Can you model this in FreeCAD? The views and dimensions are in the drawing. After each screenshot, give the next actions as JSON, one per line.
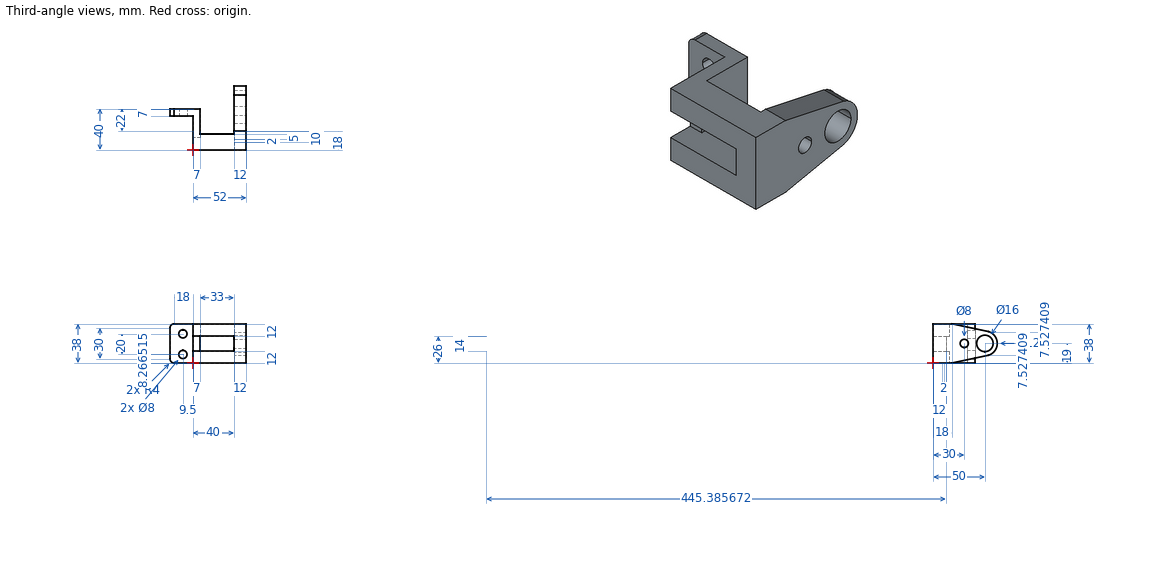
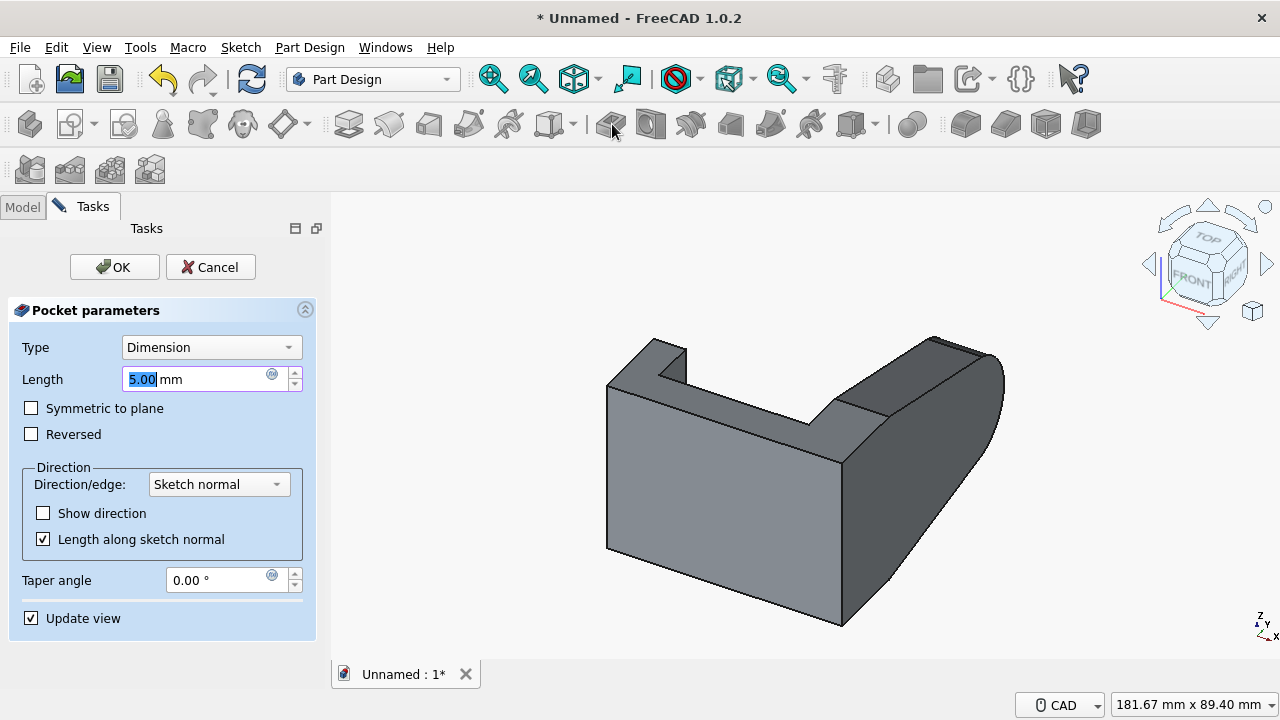
{"action": "left_click", "coordinate": [212, 348]}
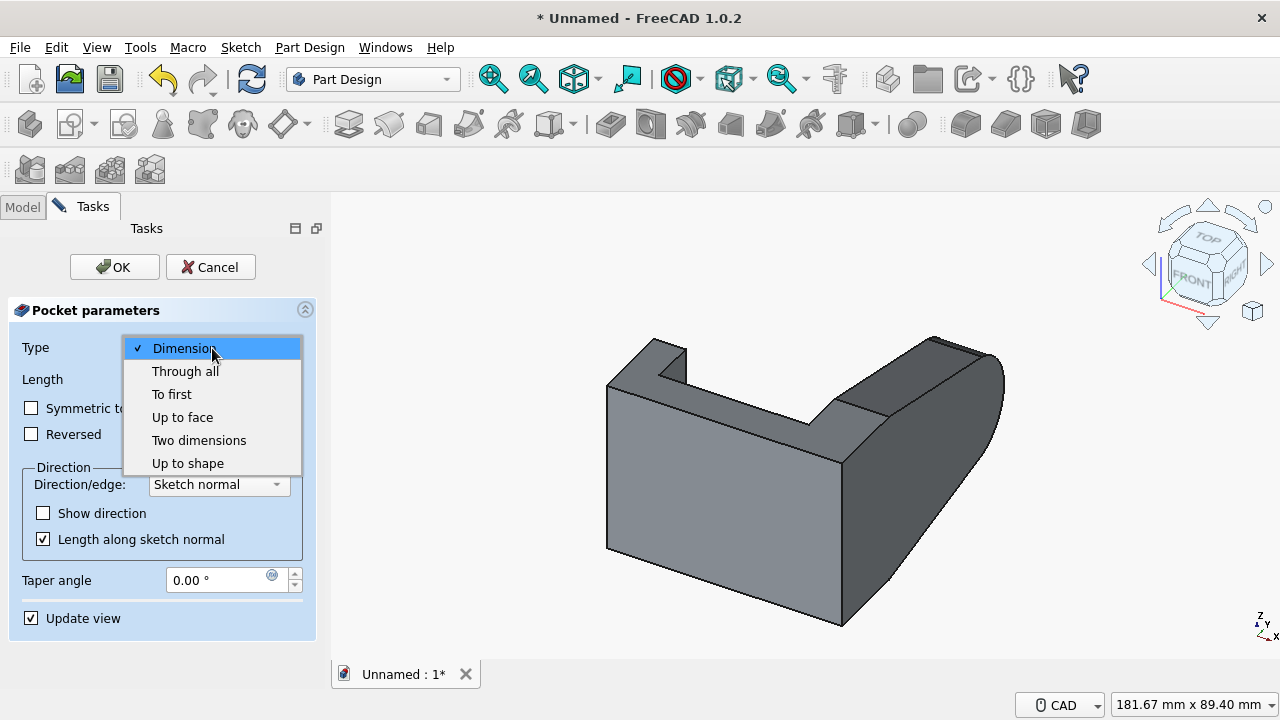
{"action": "left_click", "coordinate": [212, 440]}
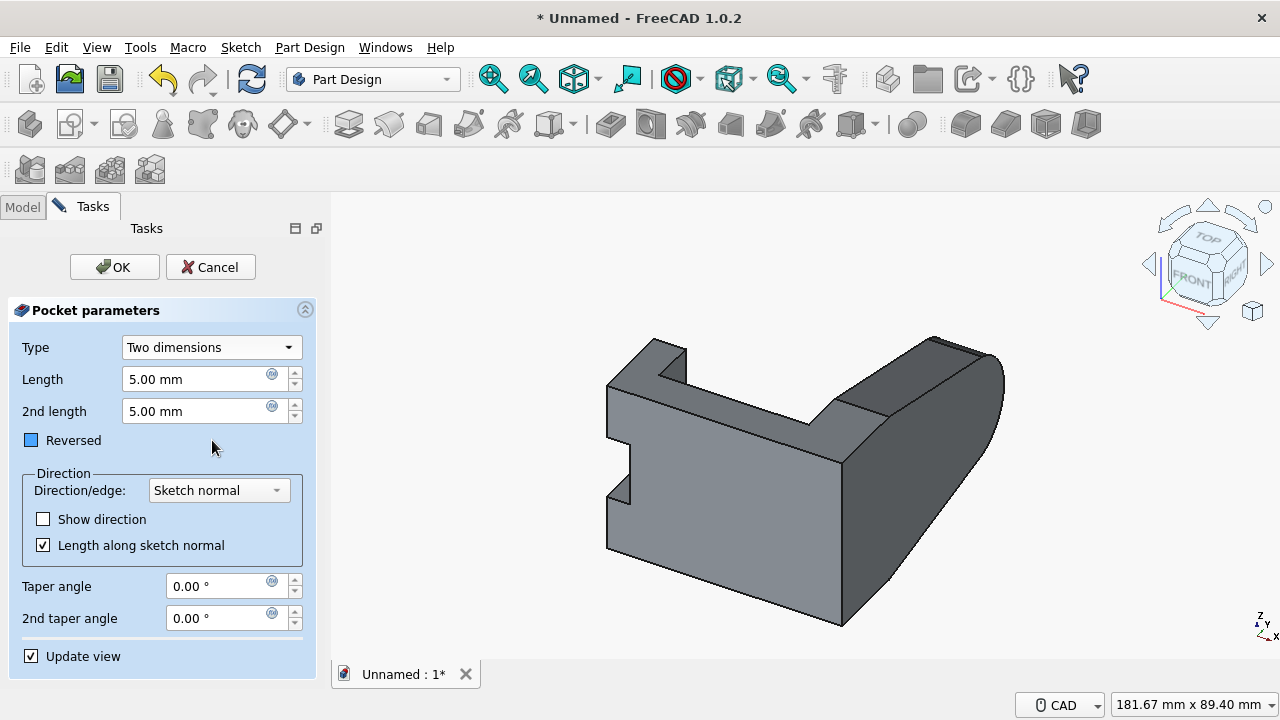
{"action": "triple_click", "coordinate": [204, 379]}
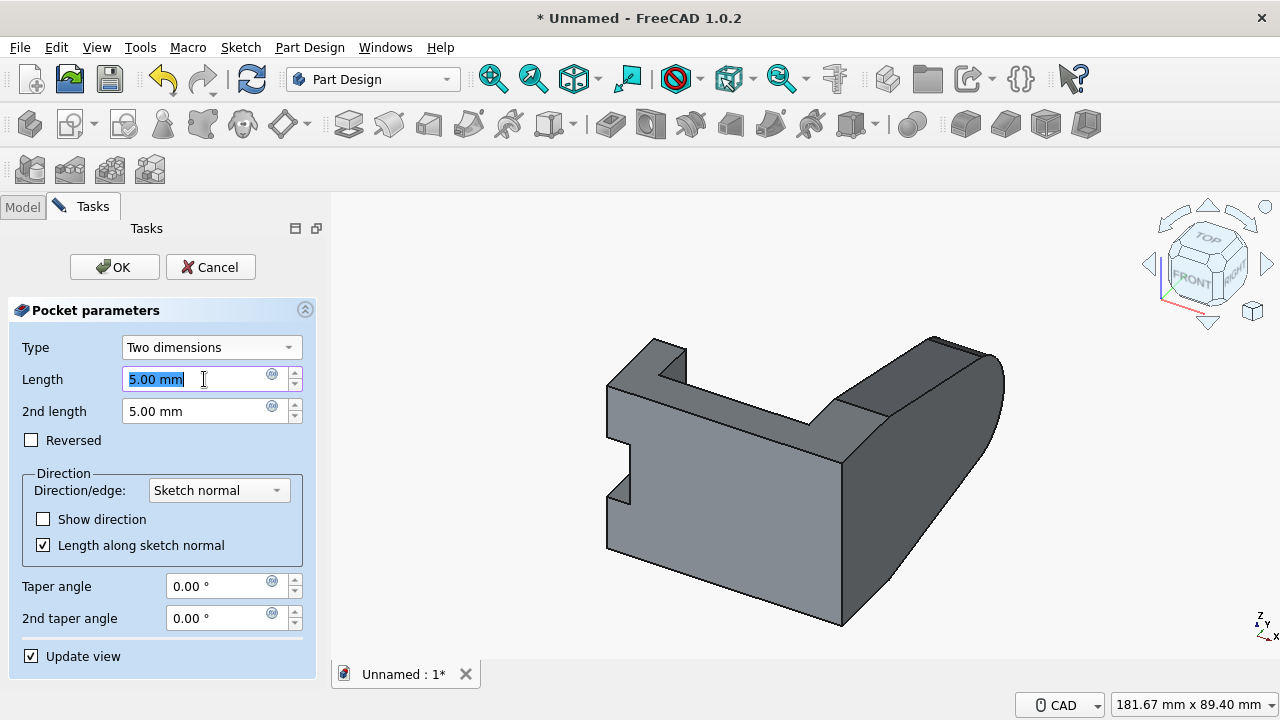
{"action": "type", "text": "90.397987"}
{"action": "key", "text": "Tab"}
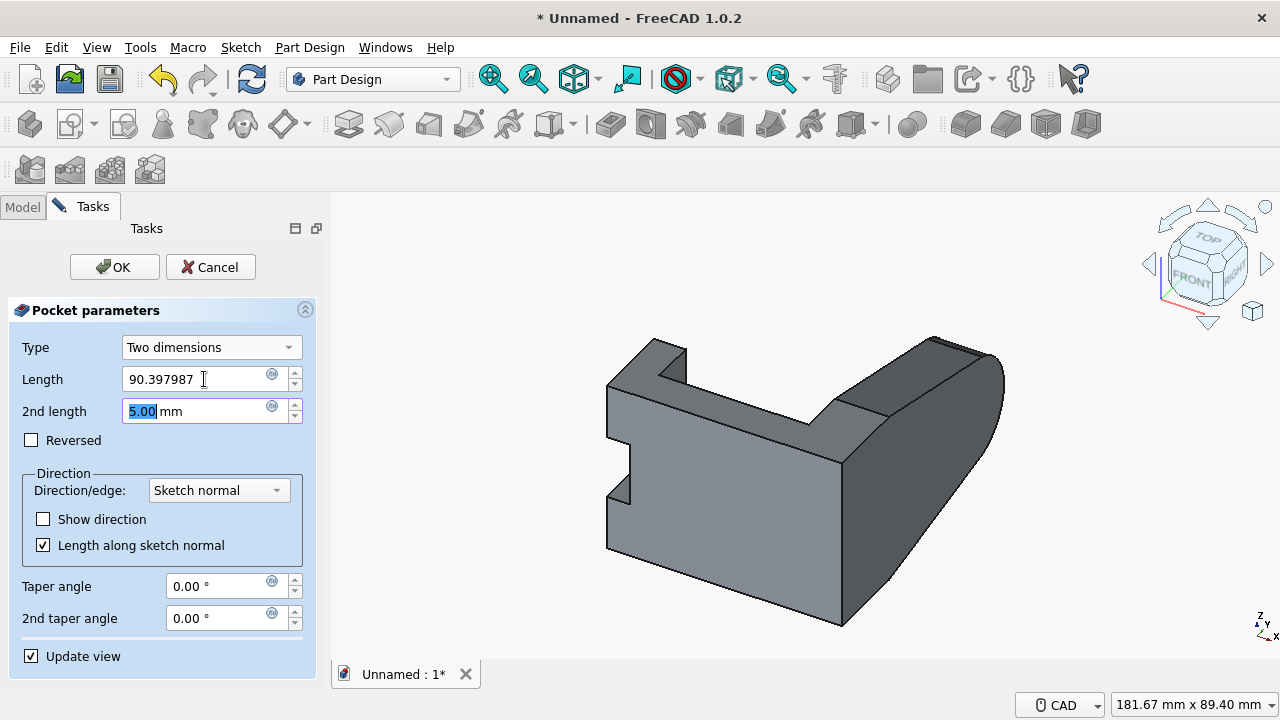
{"action": "type", "text": "40"}
{"action": "key", "text": "Tab"}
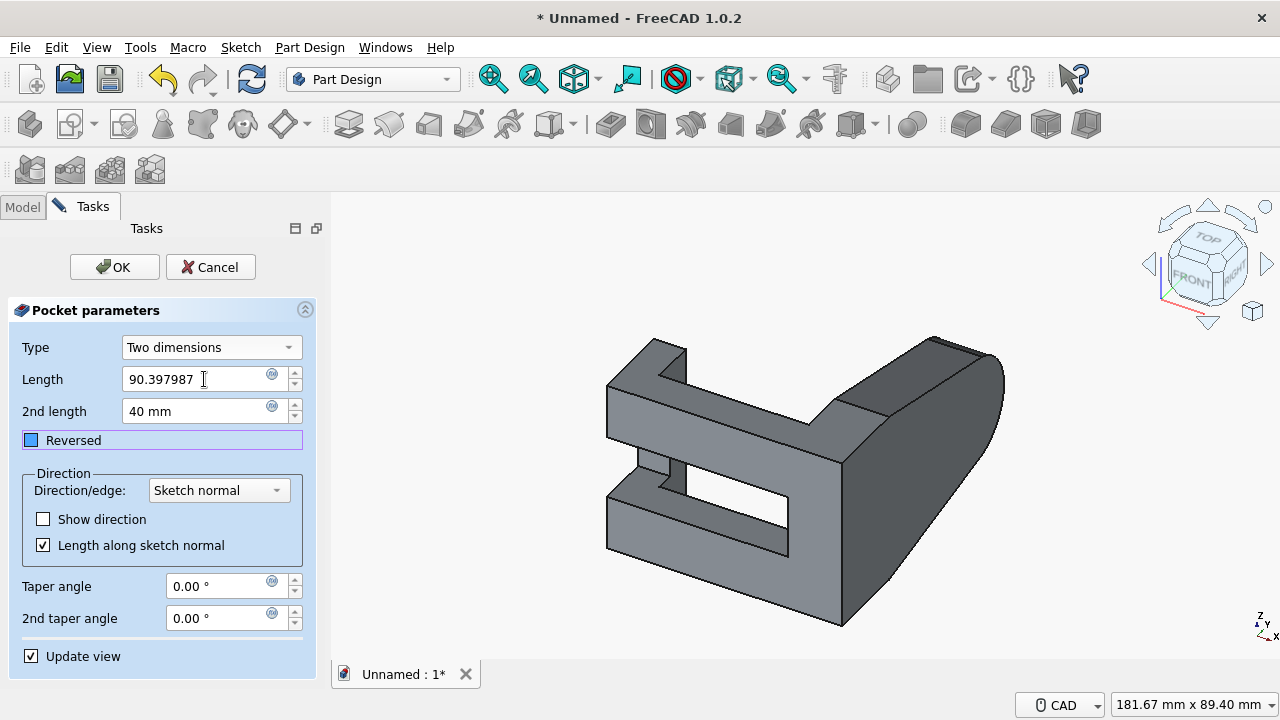
{"action": "left_click", "coordinate": [115, 267]}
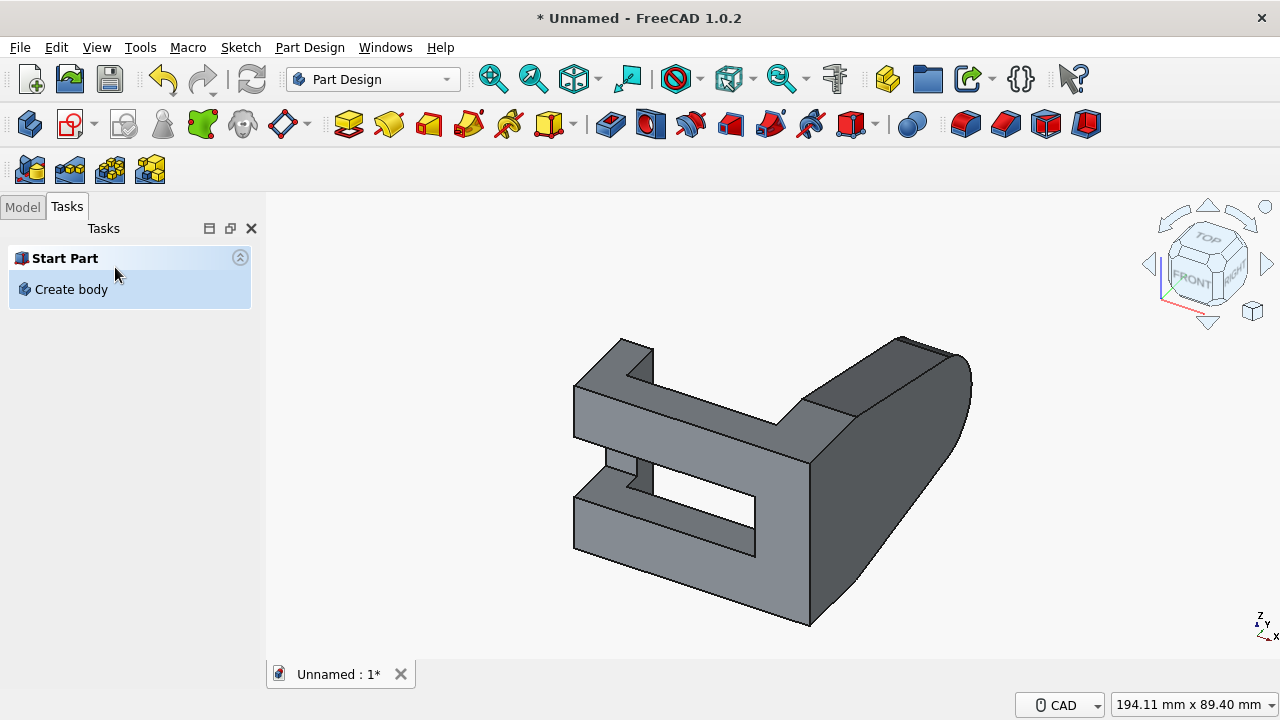
{"action": "left_click", "coordinate": [769, 436]}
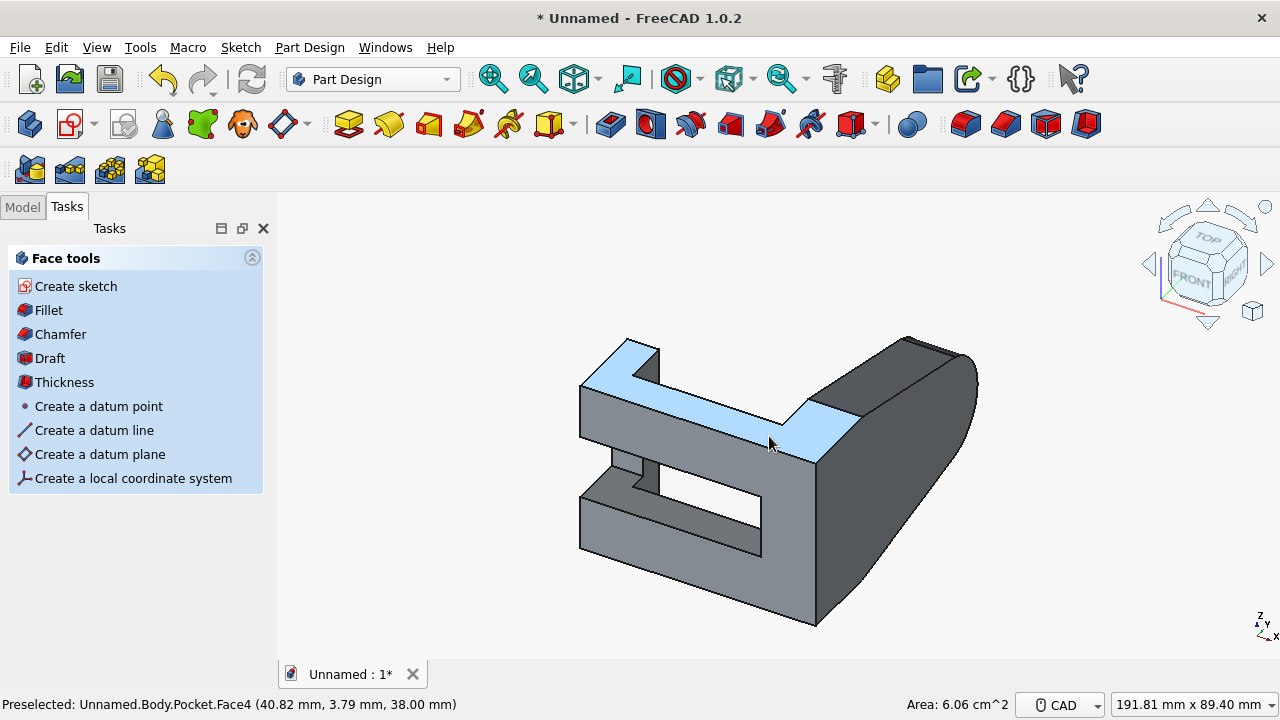
{"action": "left_click", "coordinate": [70, 124]}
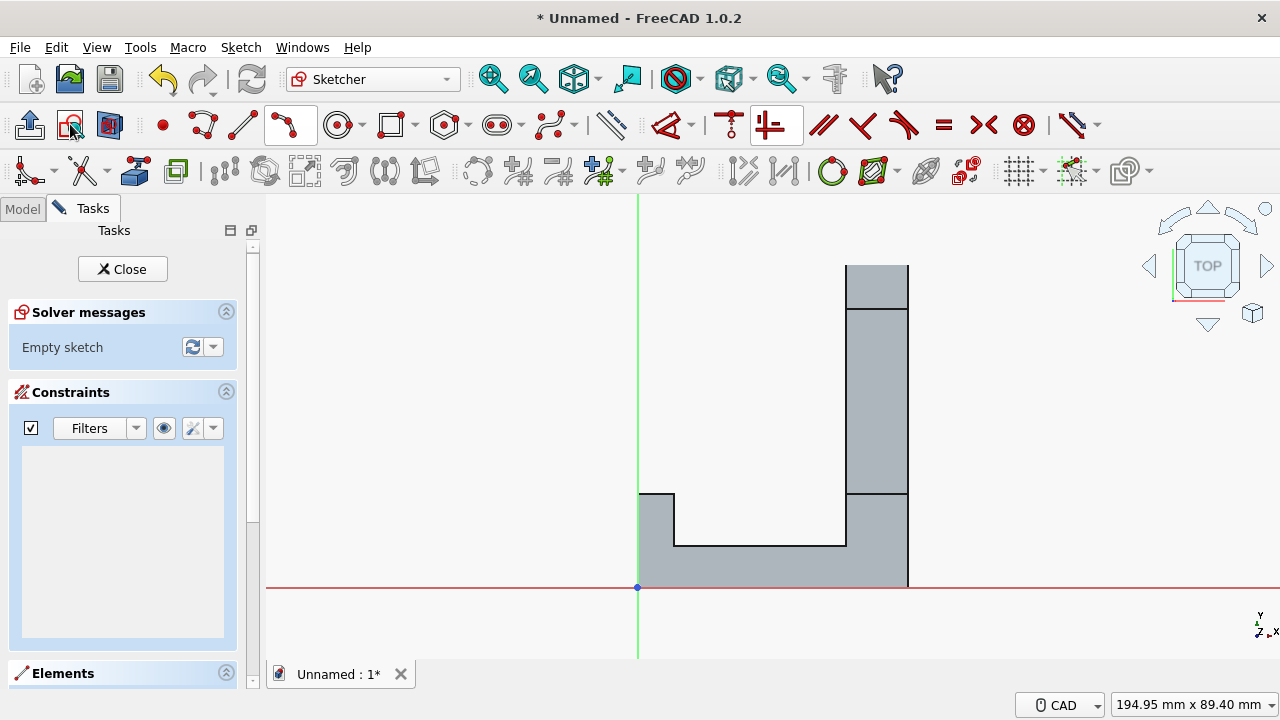
{"action": "scroll", "coordinate": [557, 600], "scroll_direction": "up", "scroll_amount": 2}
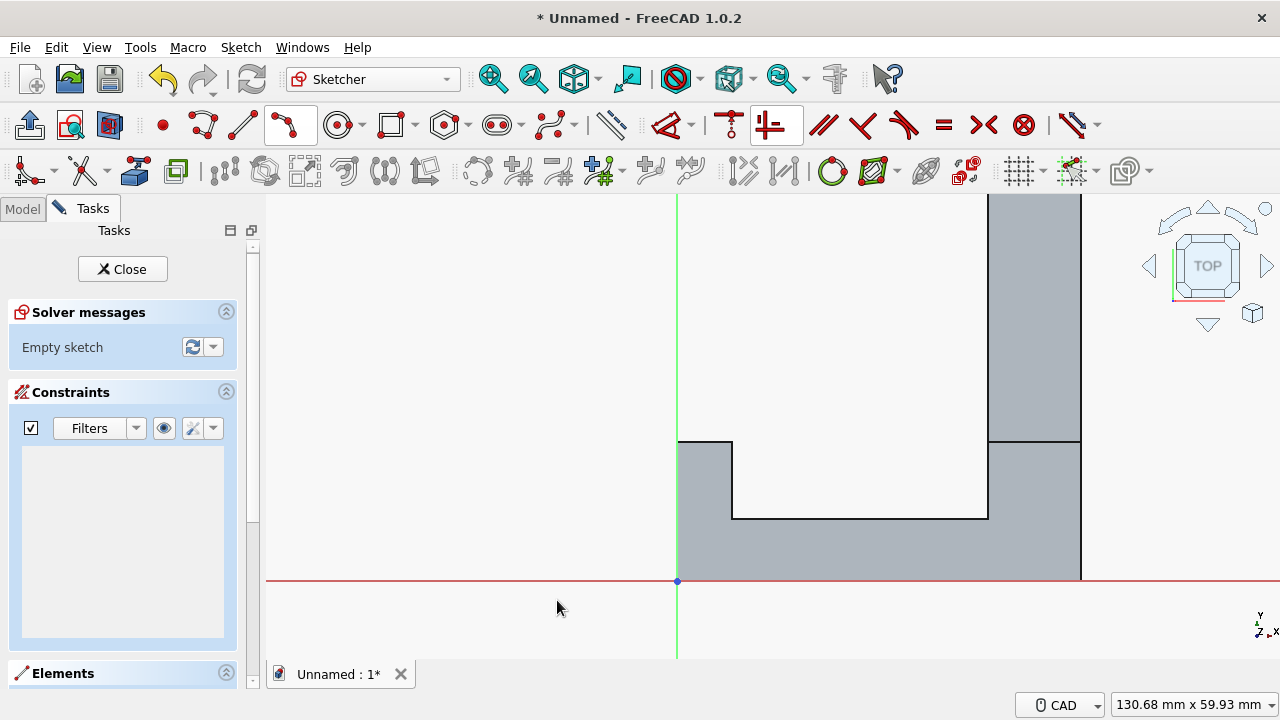
{"action": "left_click", "coordinate": [392, 126]}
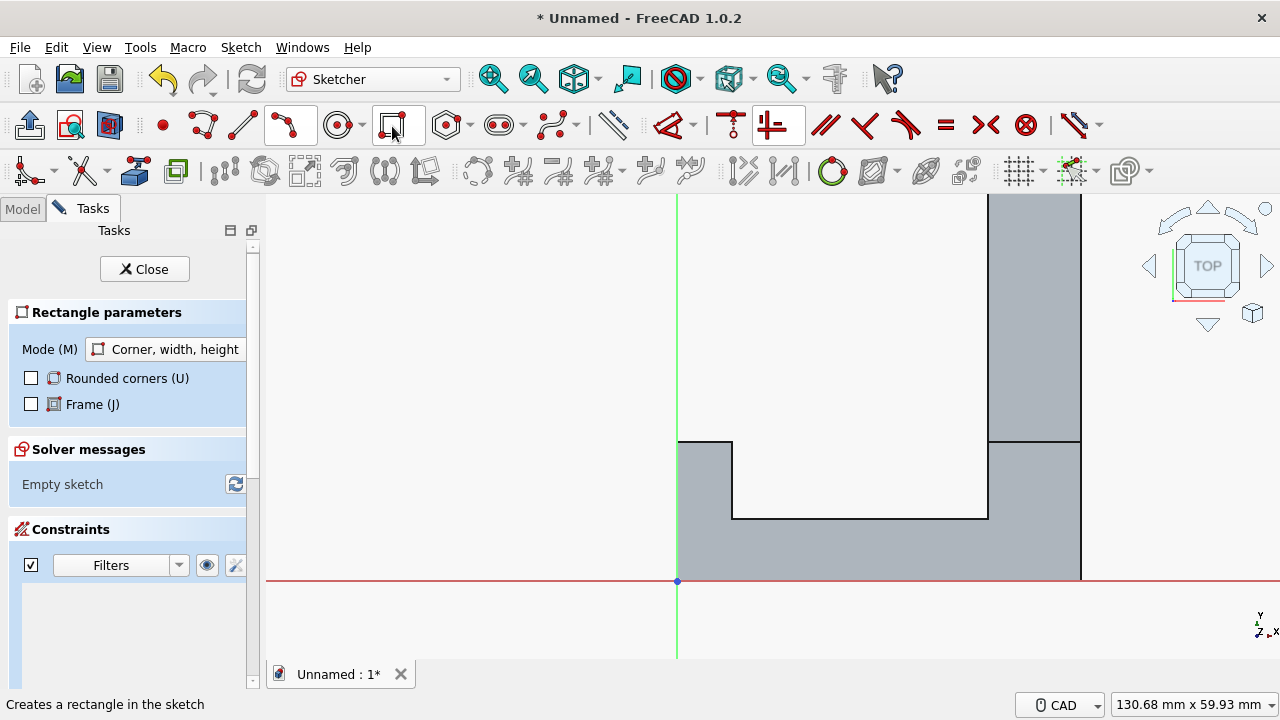
{"action": "left_click", "coordinate": [677, 271]}
{"action": "left_click", "coordinate": [732, 442]}
{"action": "key", "text": "Escape"}